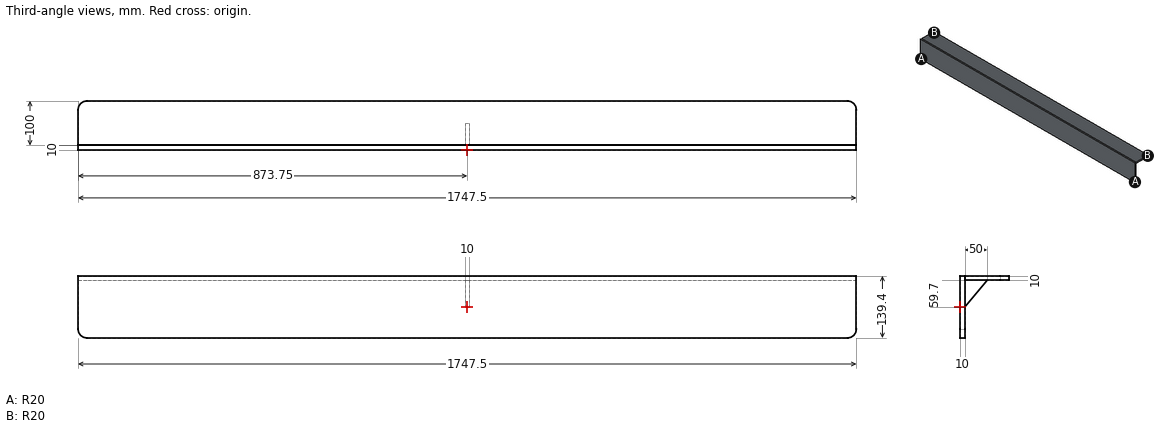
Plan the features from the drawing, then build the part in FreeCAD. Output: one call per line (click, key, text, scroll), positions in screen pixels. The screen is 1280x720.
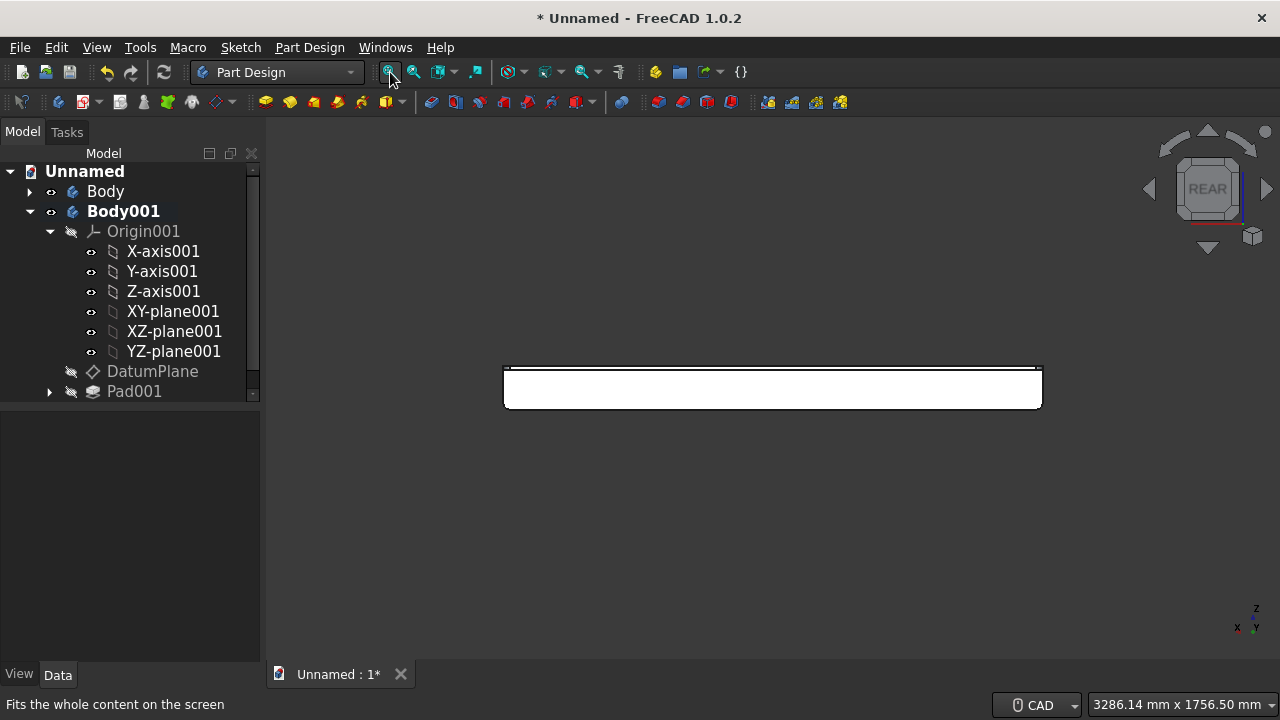
click(60, 102)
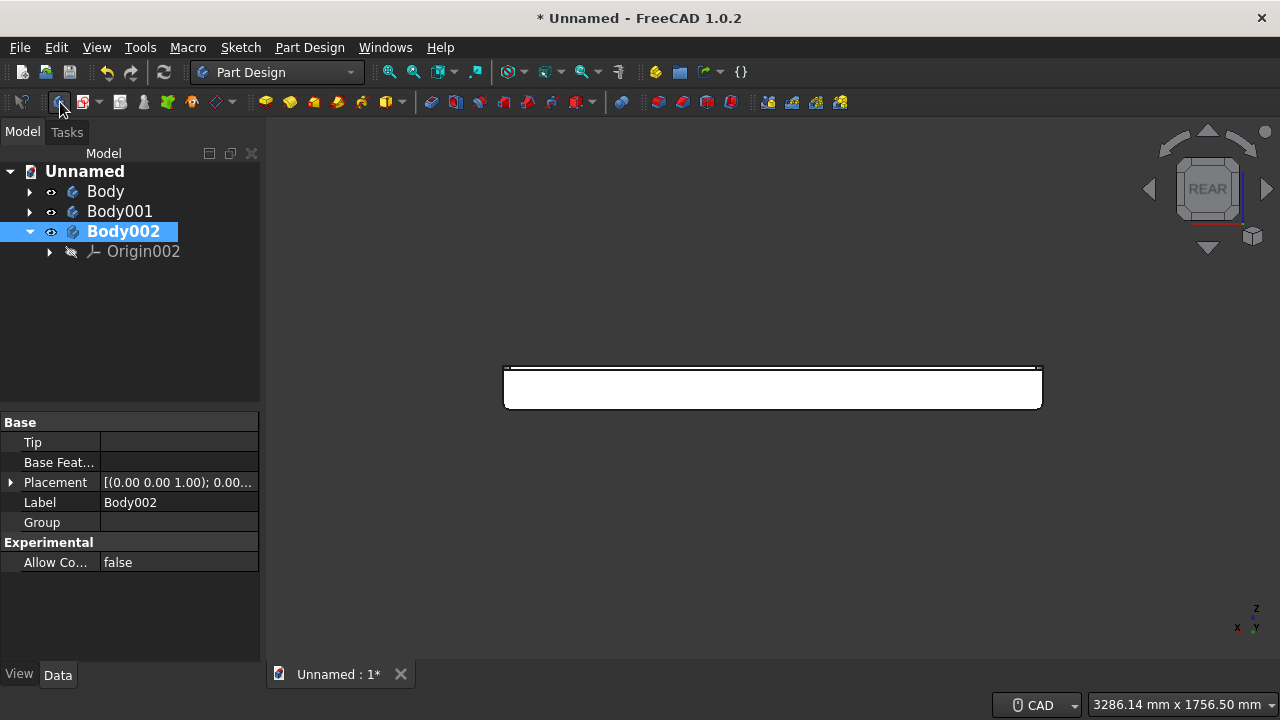
click(306, 619)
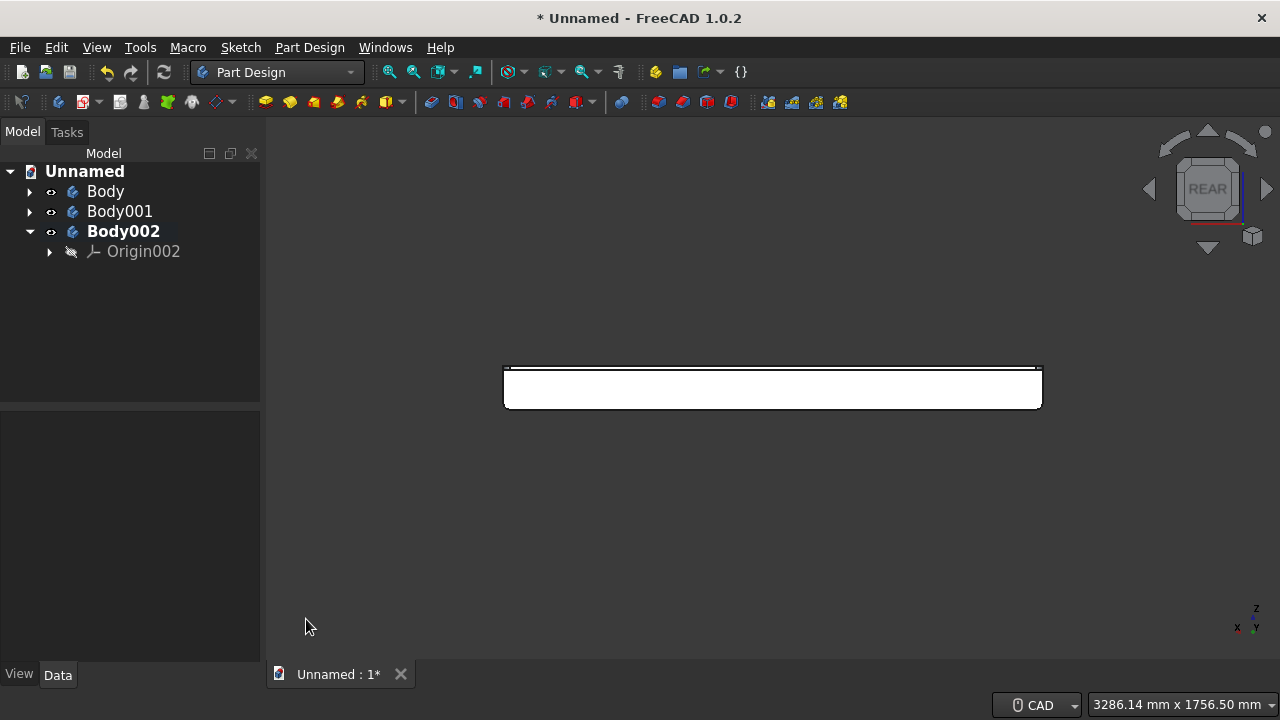
click(84, 102)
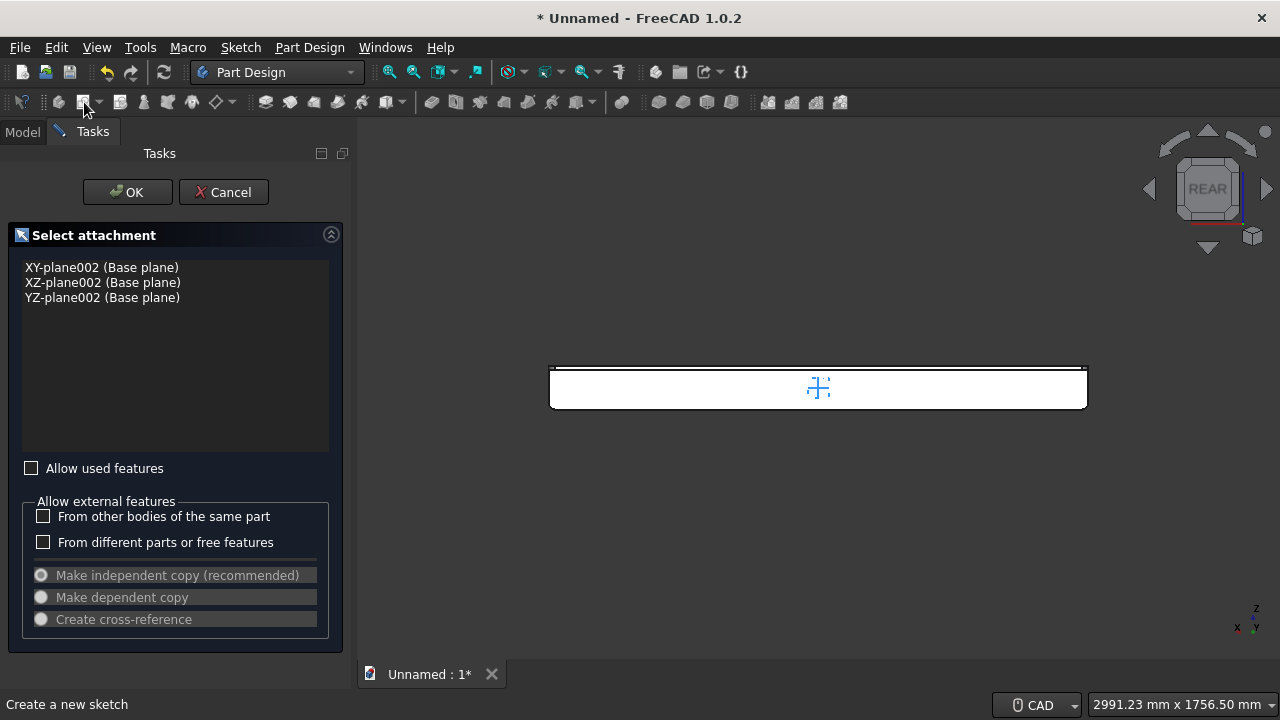
click(82, 298)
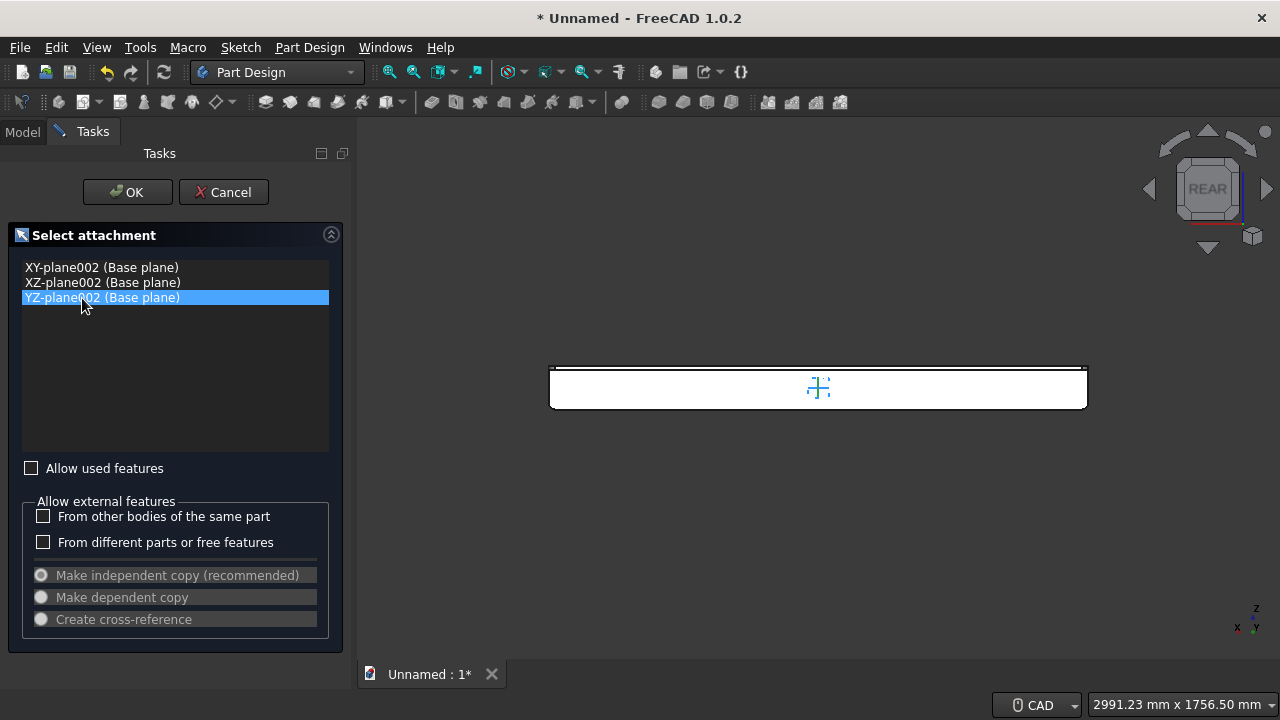
click(128, 192)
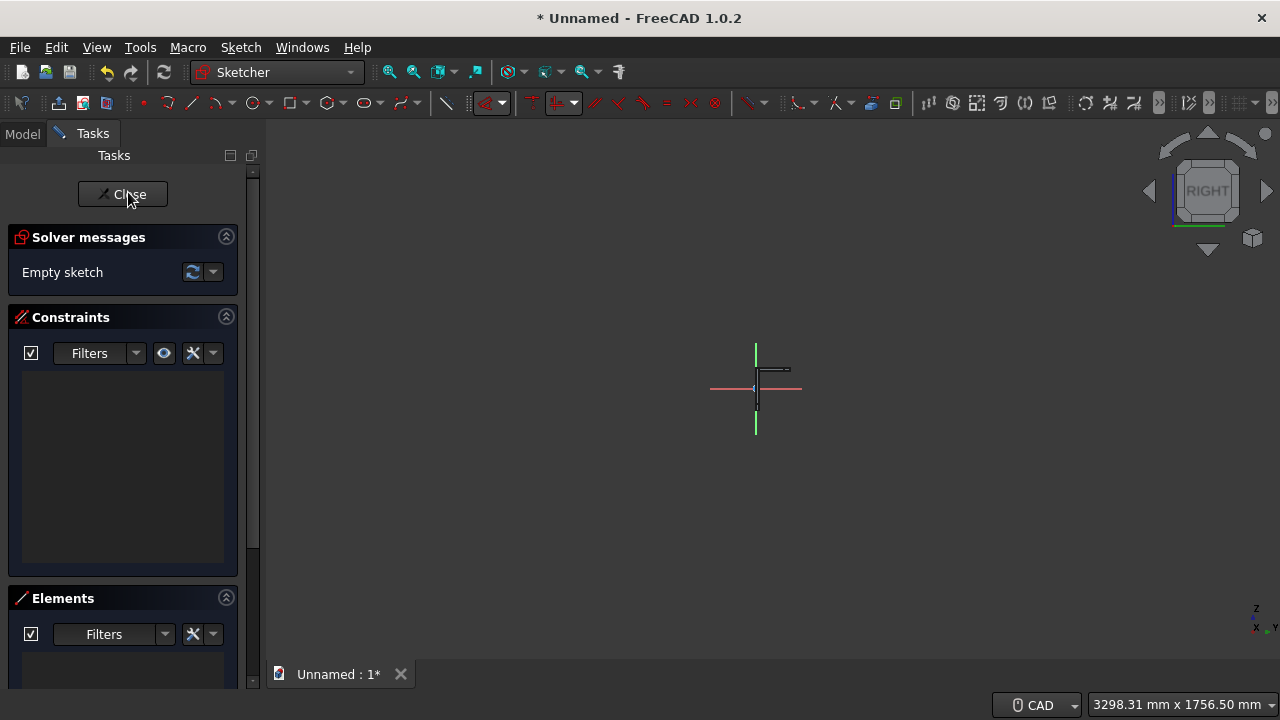
scroll(769, 379, up, 15)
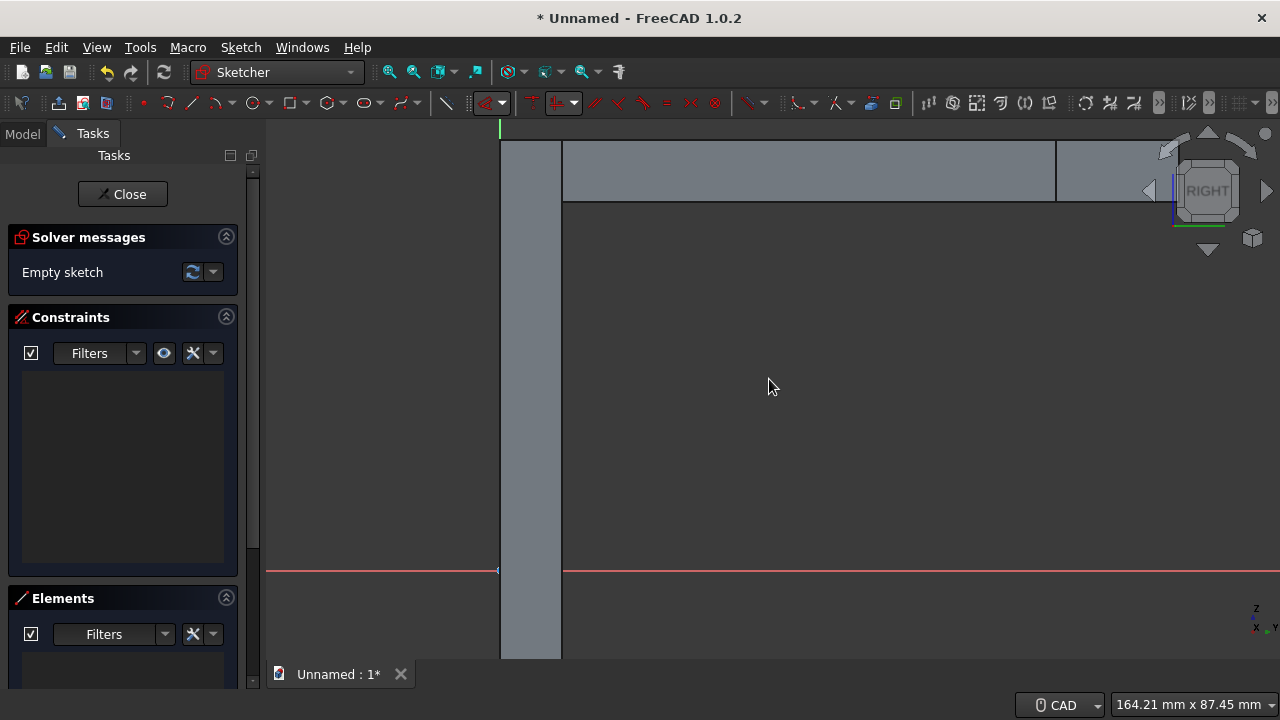
click(168, 104)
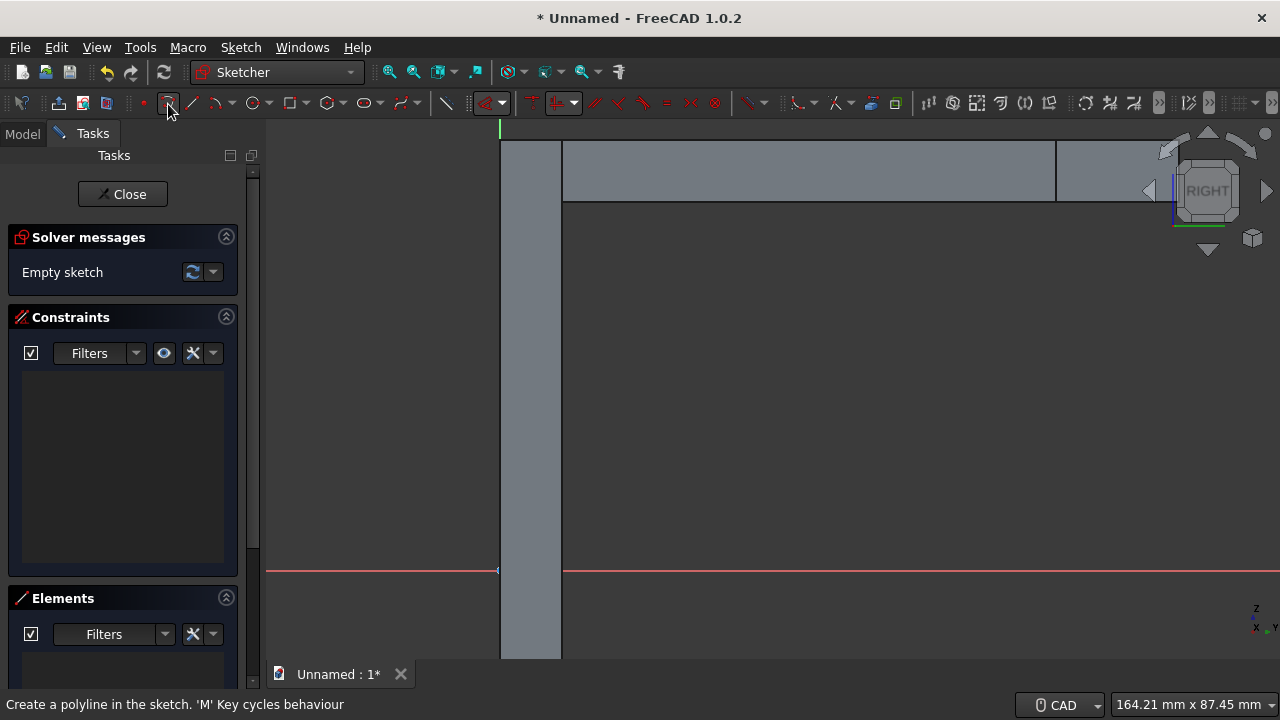
click(562, 571)
click(871, 202)
click(562, 202)
click(562, 571)
key(Escape)
key(Escape)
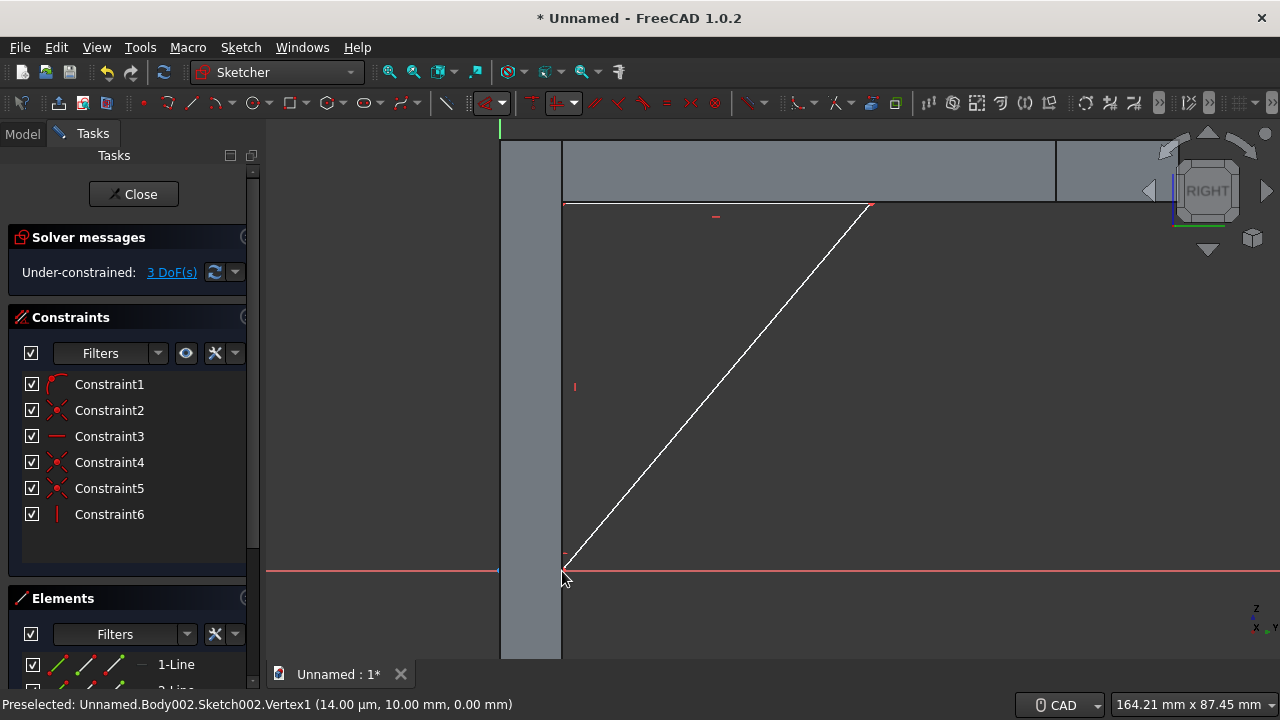
click(778, 203)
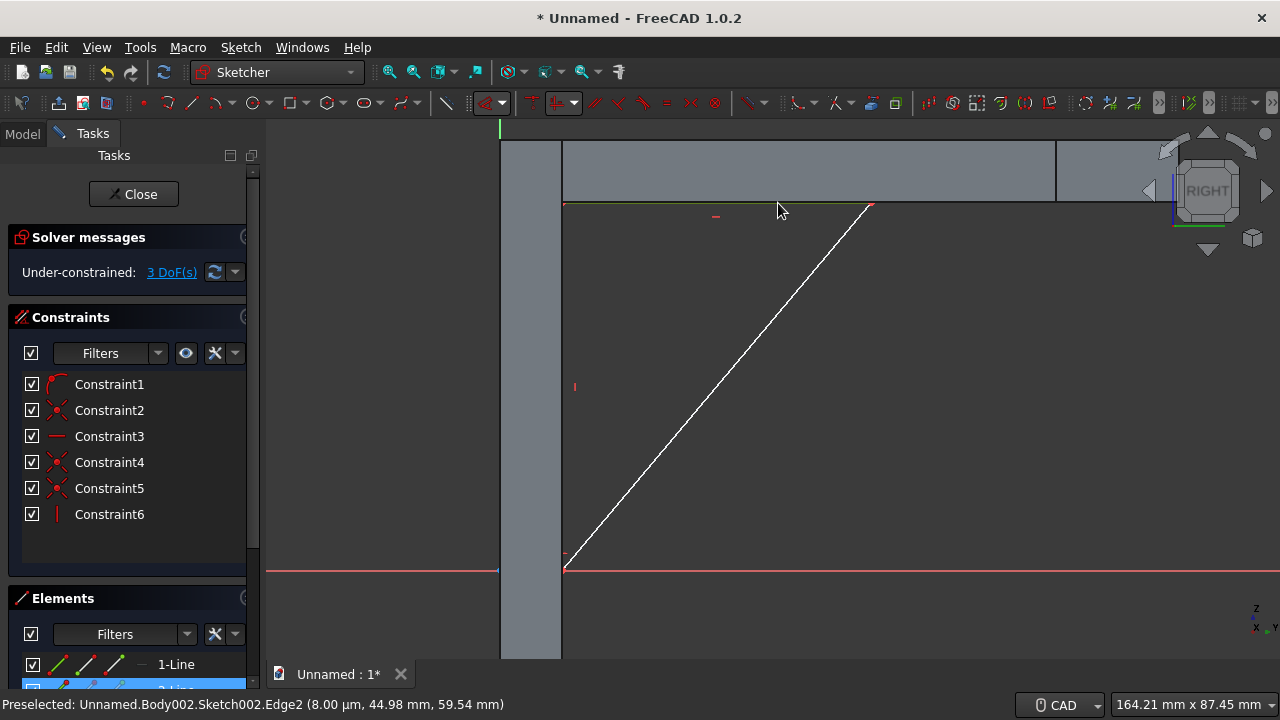
key(l)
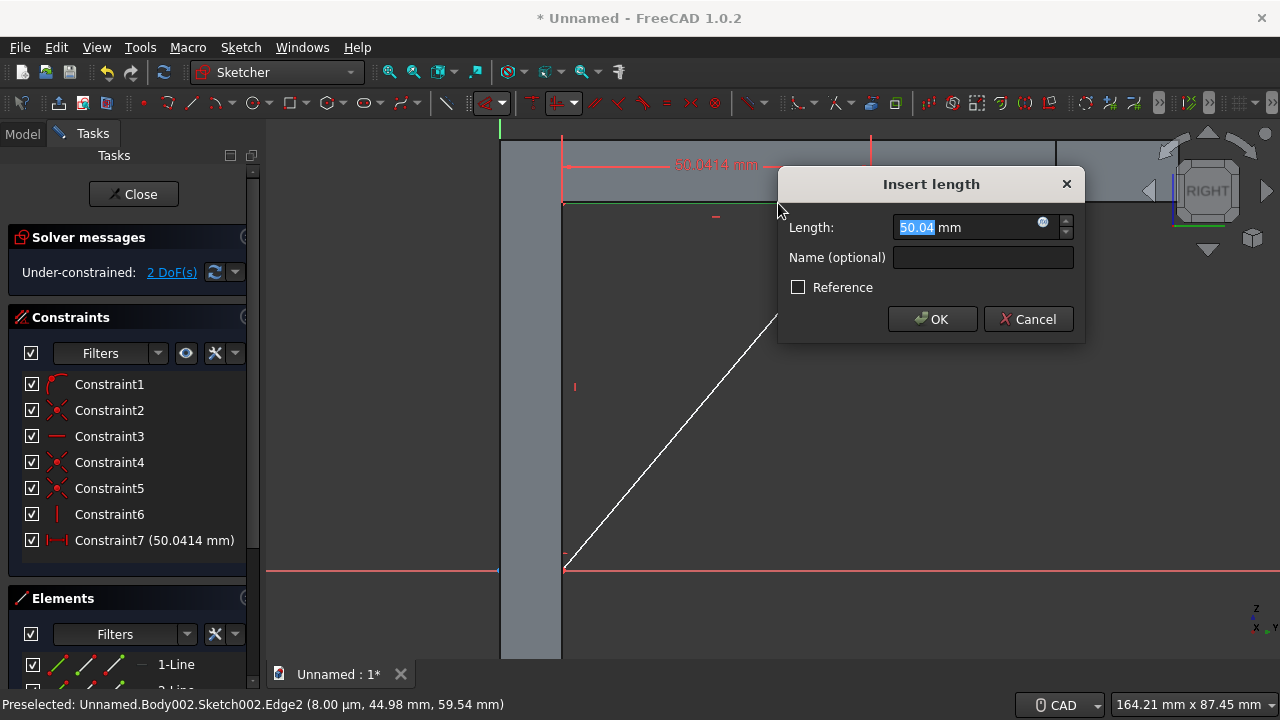
text(50)
key(Return)